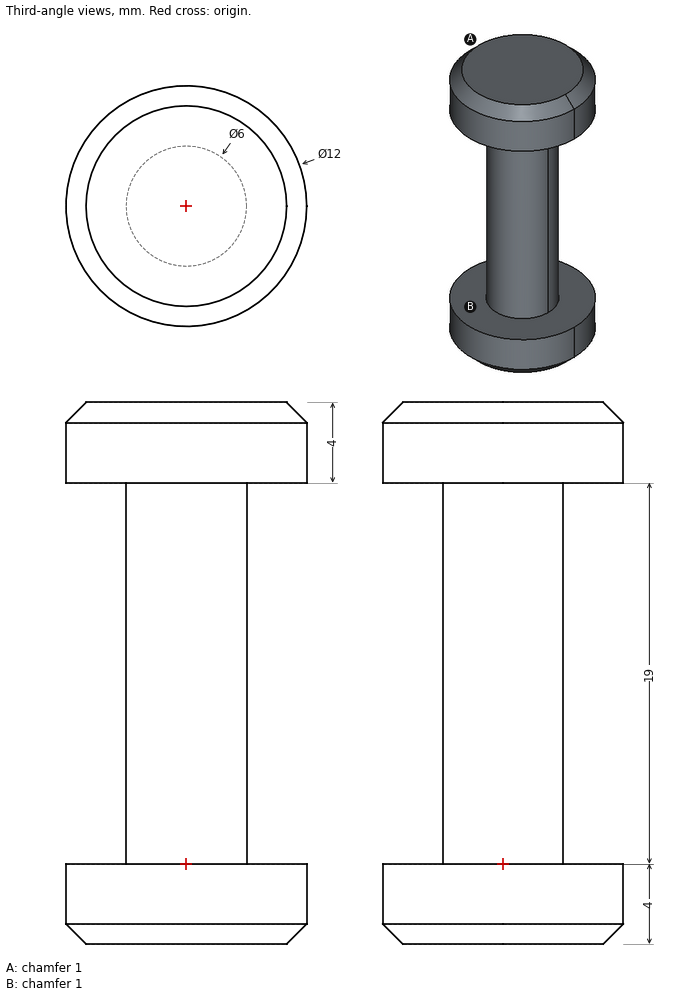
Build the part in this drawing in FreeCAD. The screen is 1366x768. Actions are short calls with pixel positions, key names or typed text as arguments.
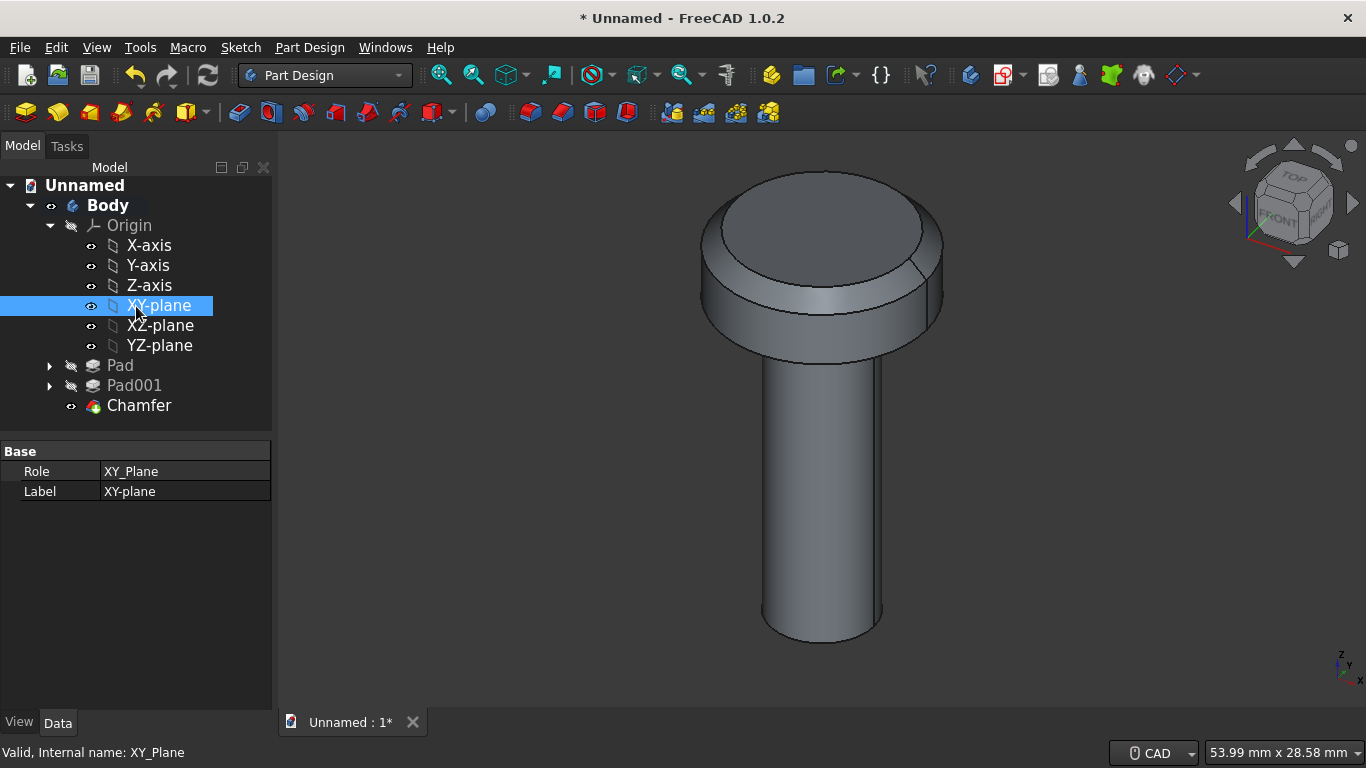
click(1176, 76)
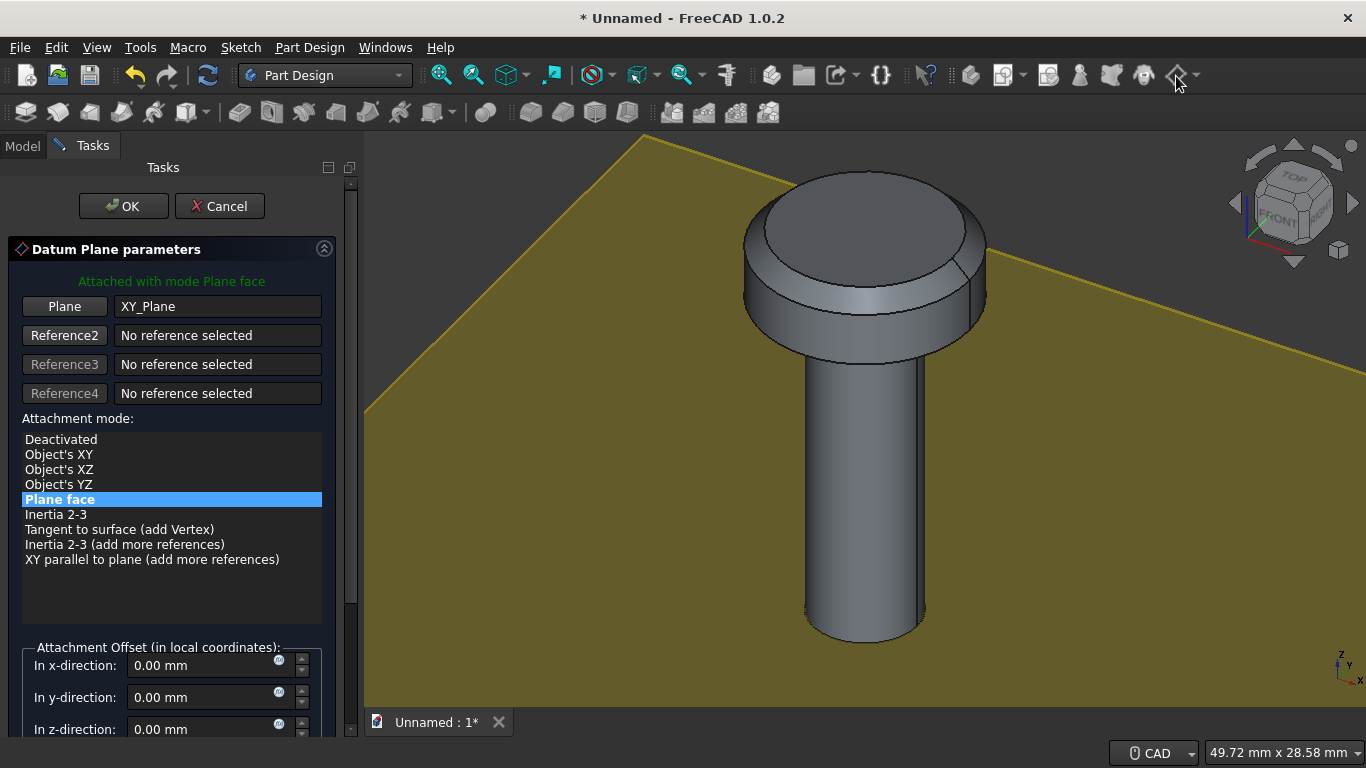
scroll(351, 456, down, 2)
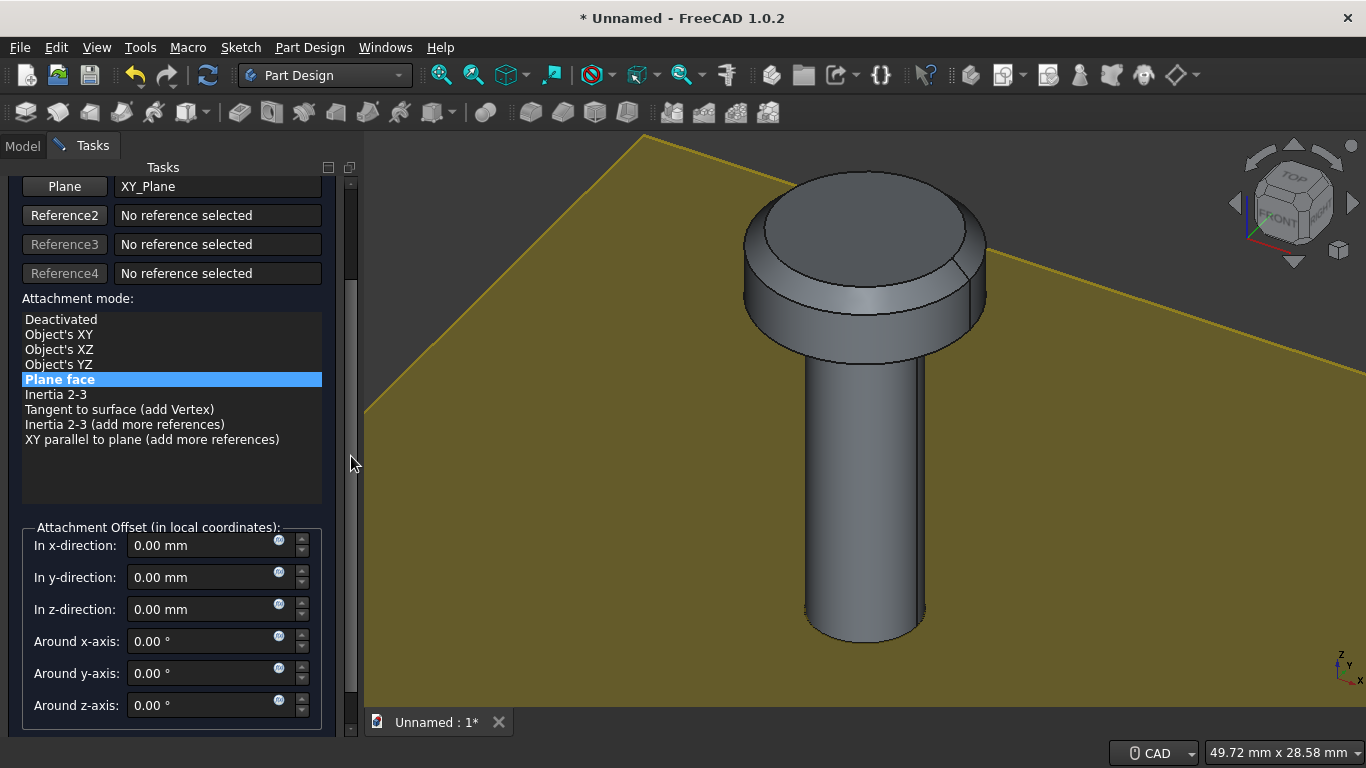
triple_click(210, 609)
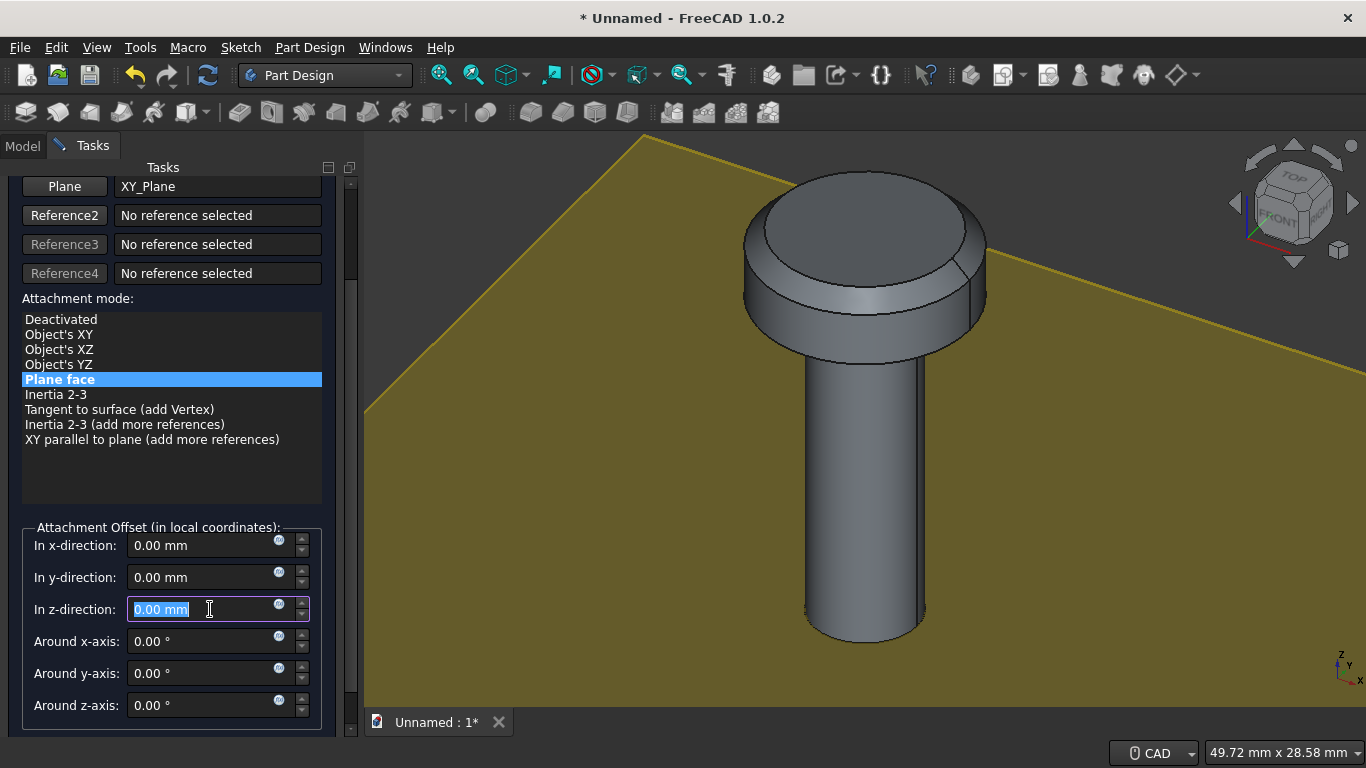
text(-4)
key(Tab)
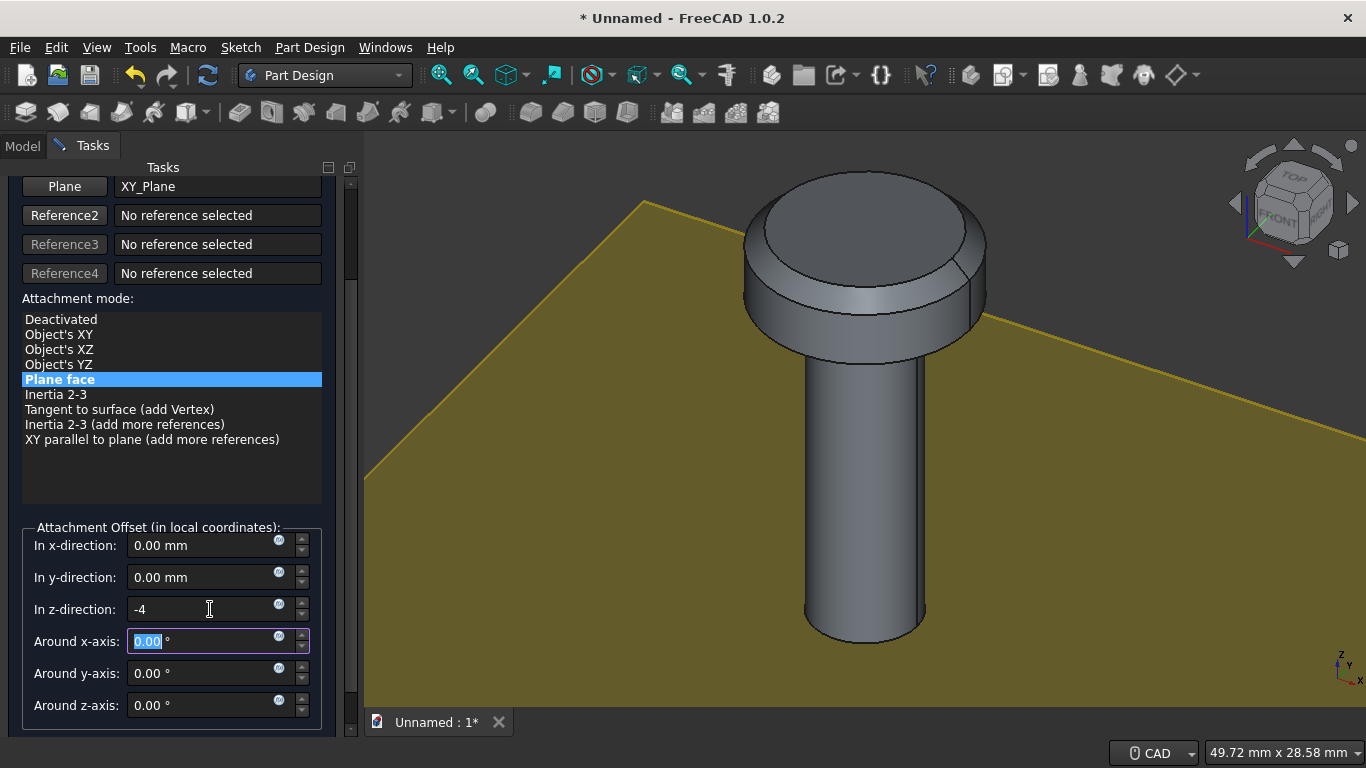
scroll(351, 456, up, 3)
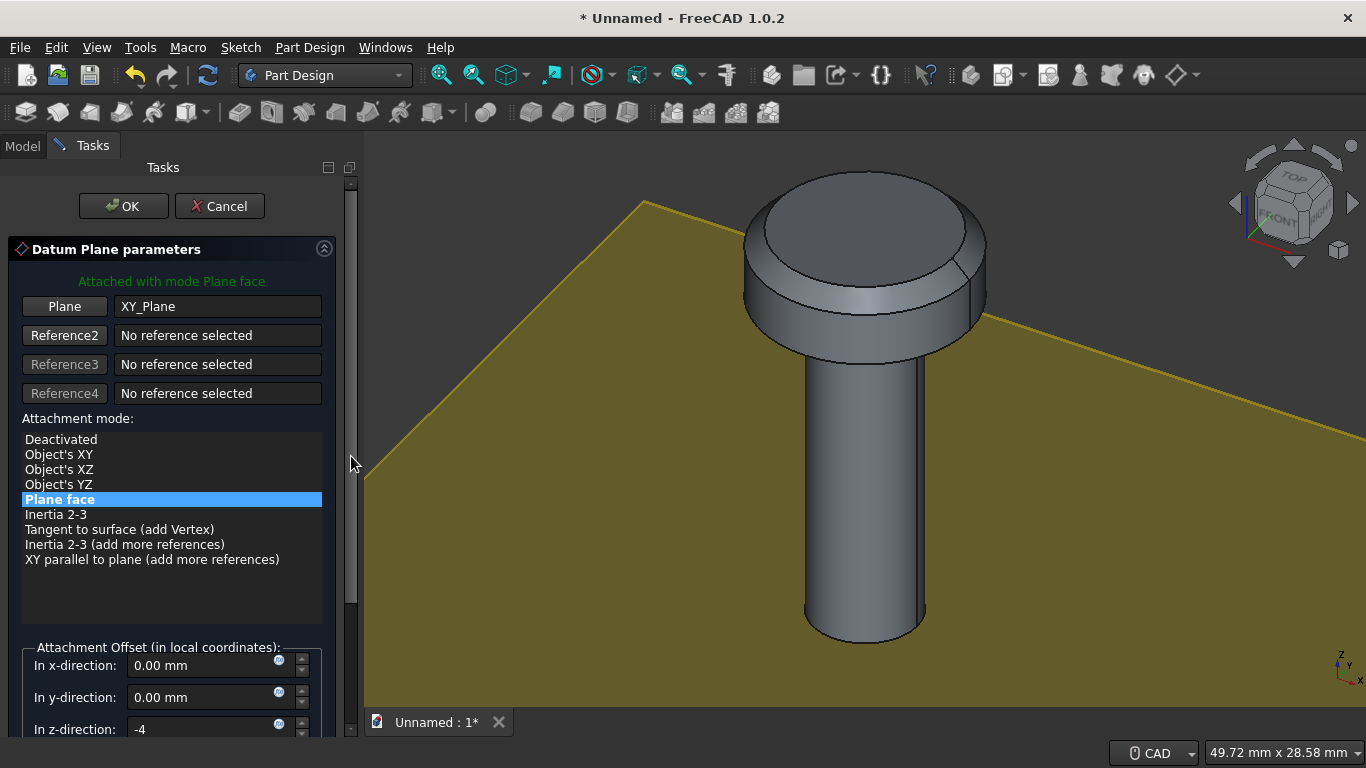
click(124, 206)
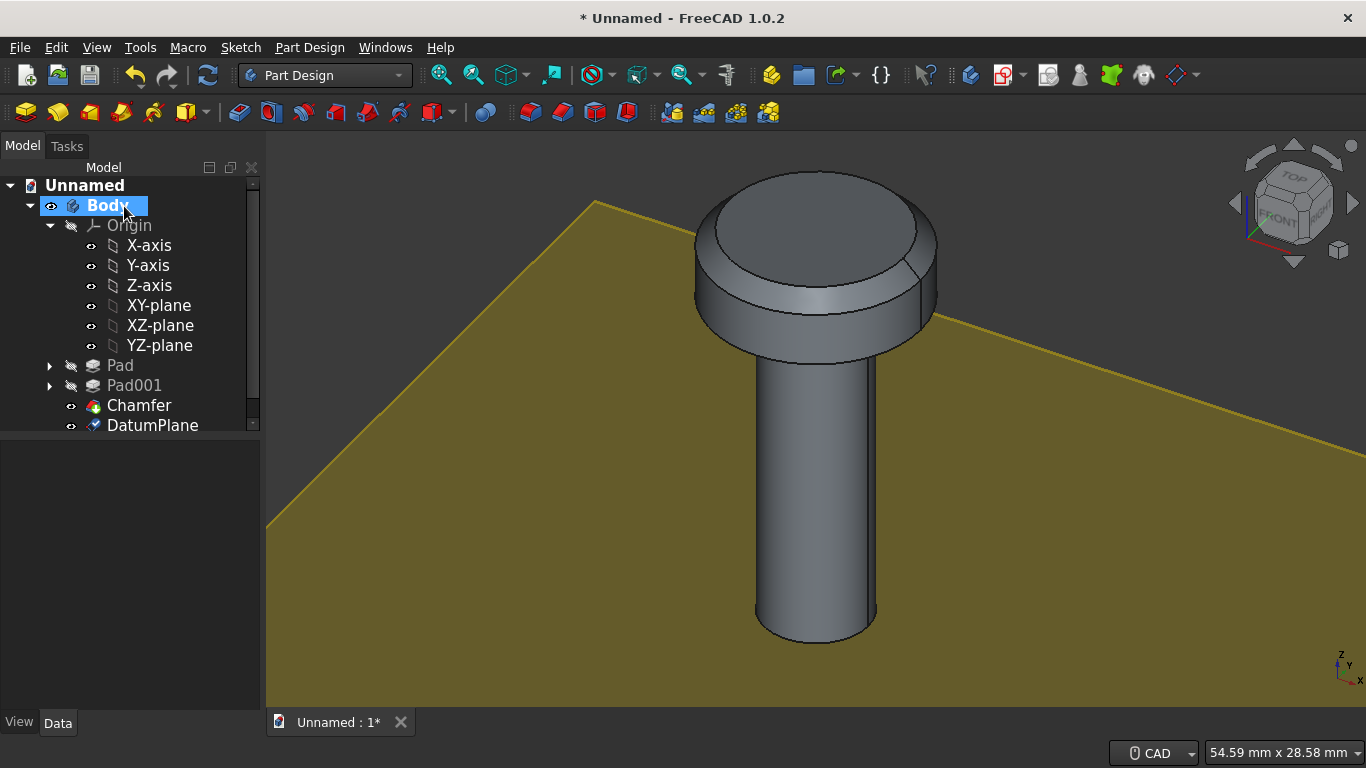
click(116, 426)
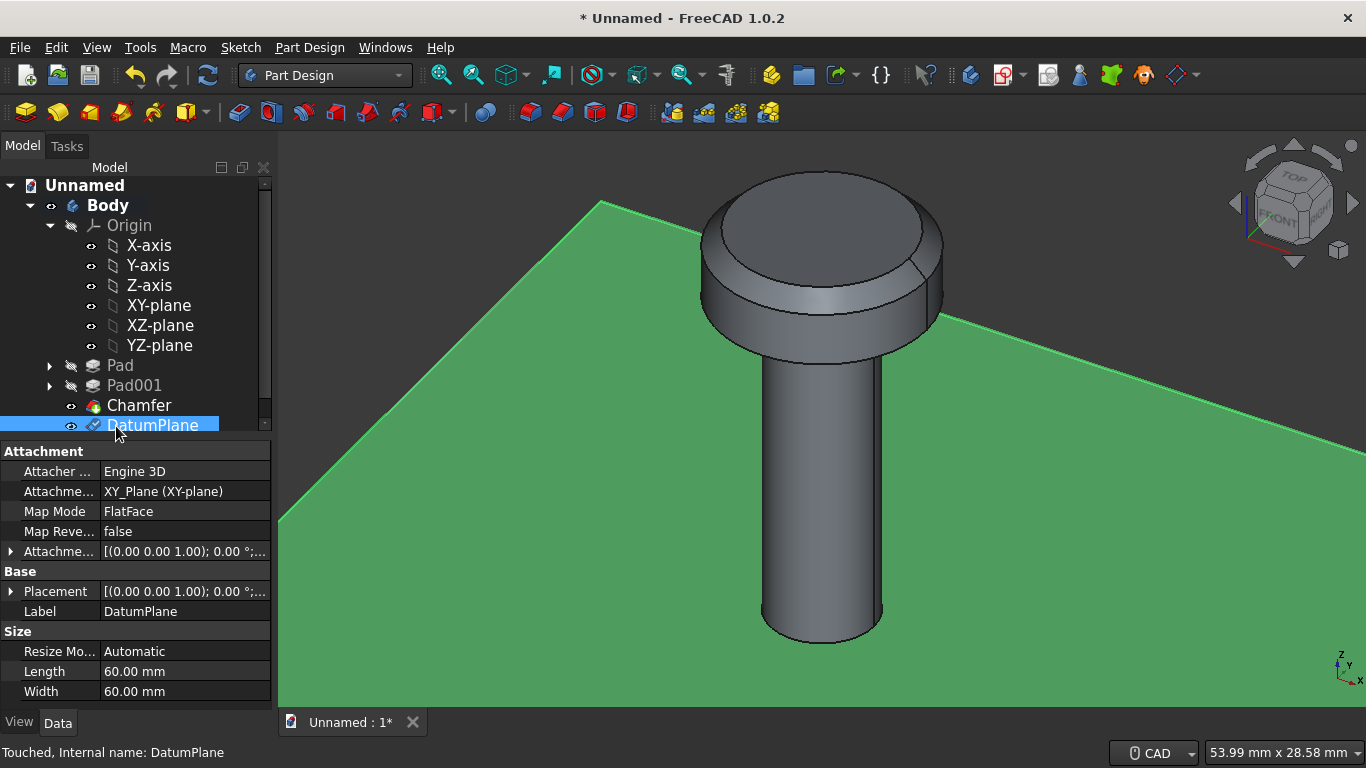
click(1004, 76)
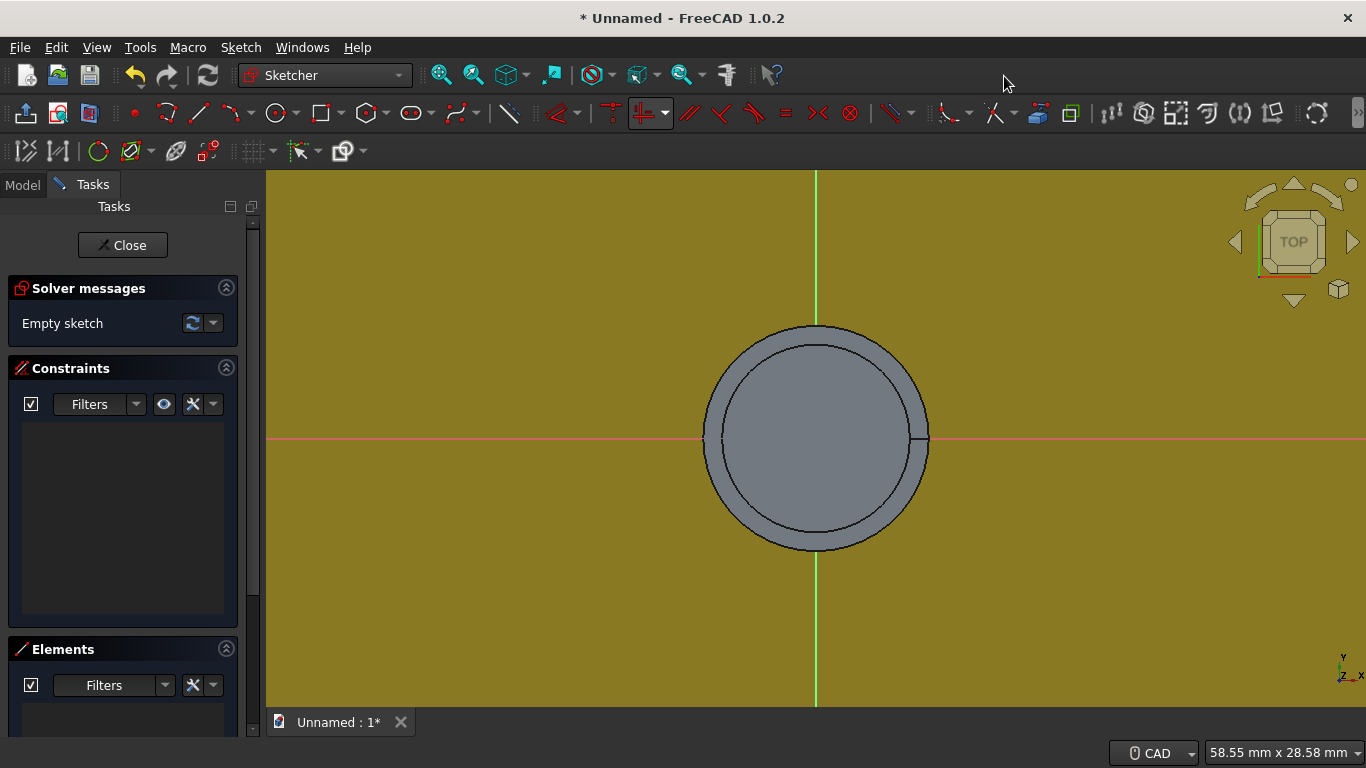
click(90, 114)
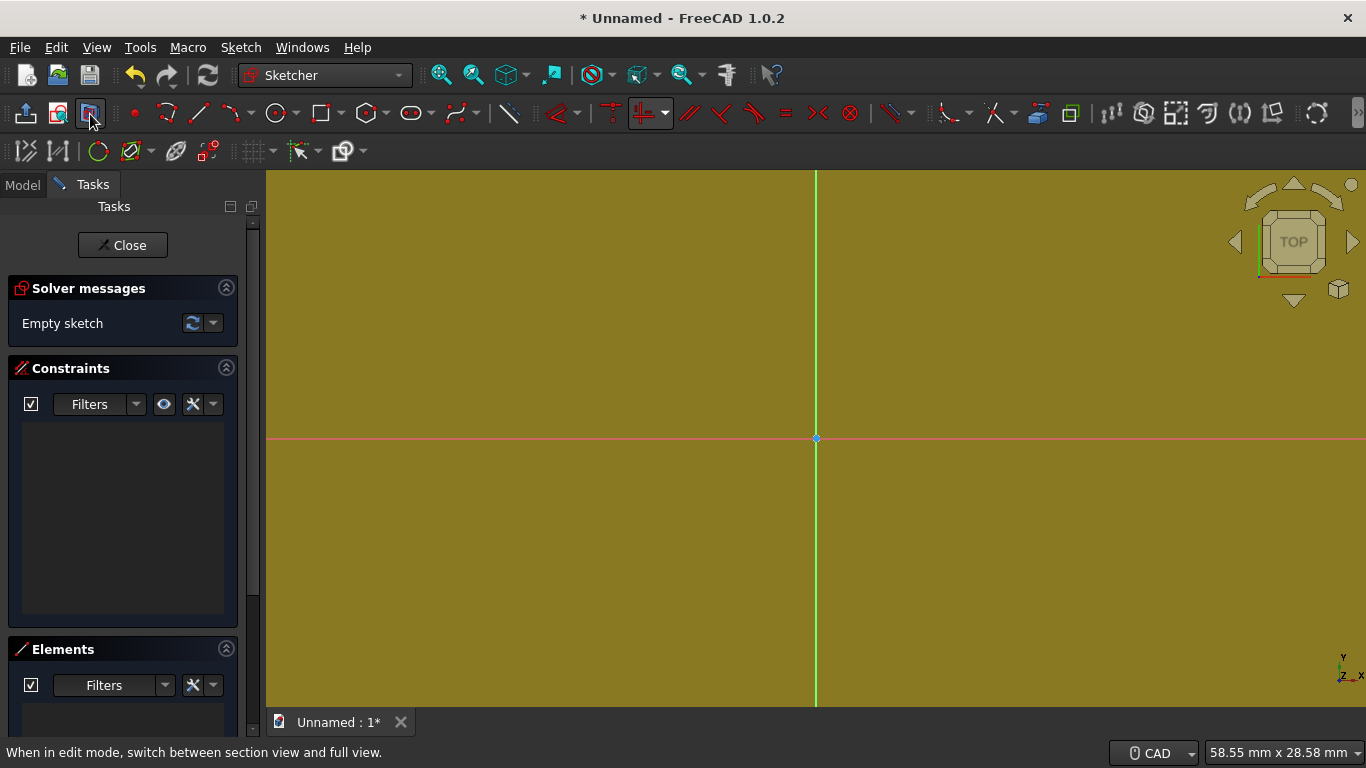
scroll(955, 439, up, 2)